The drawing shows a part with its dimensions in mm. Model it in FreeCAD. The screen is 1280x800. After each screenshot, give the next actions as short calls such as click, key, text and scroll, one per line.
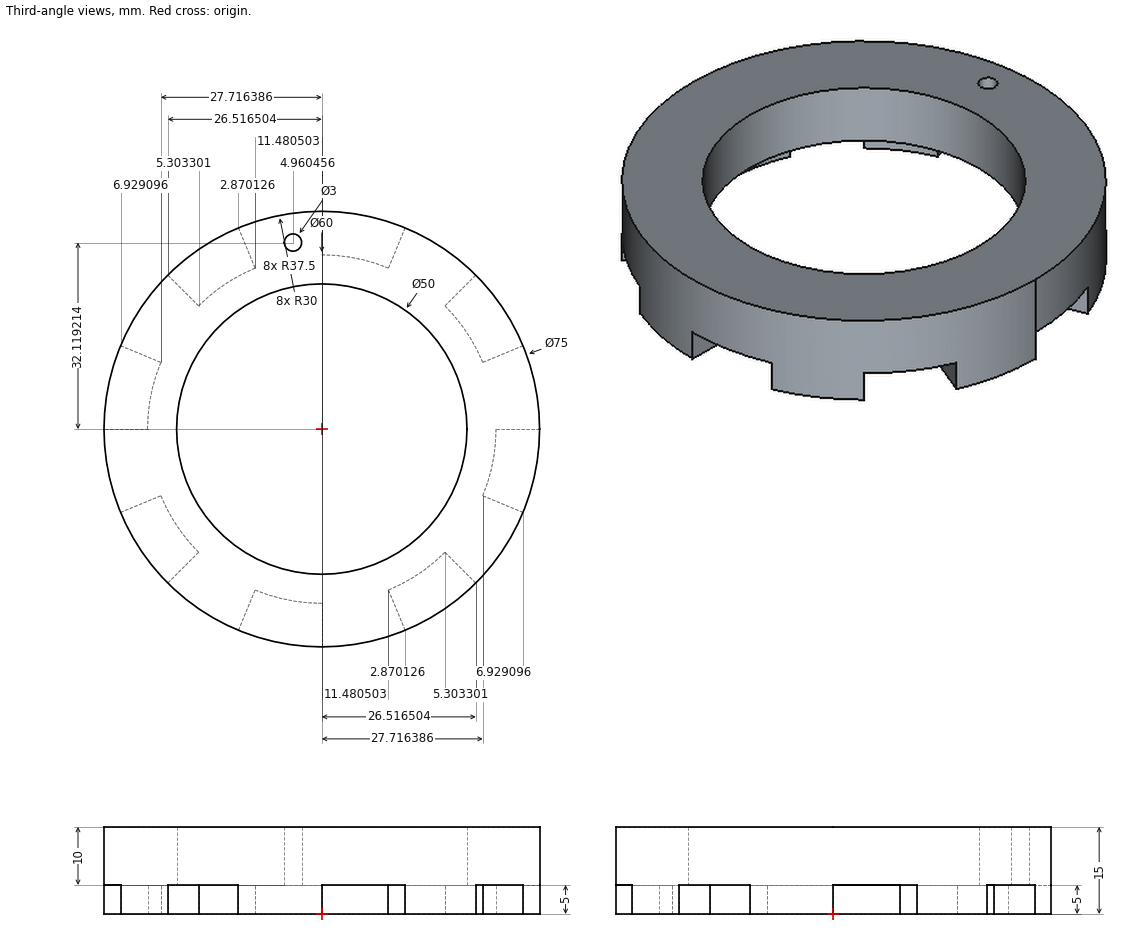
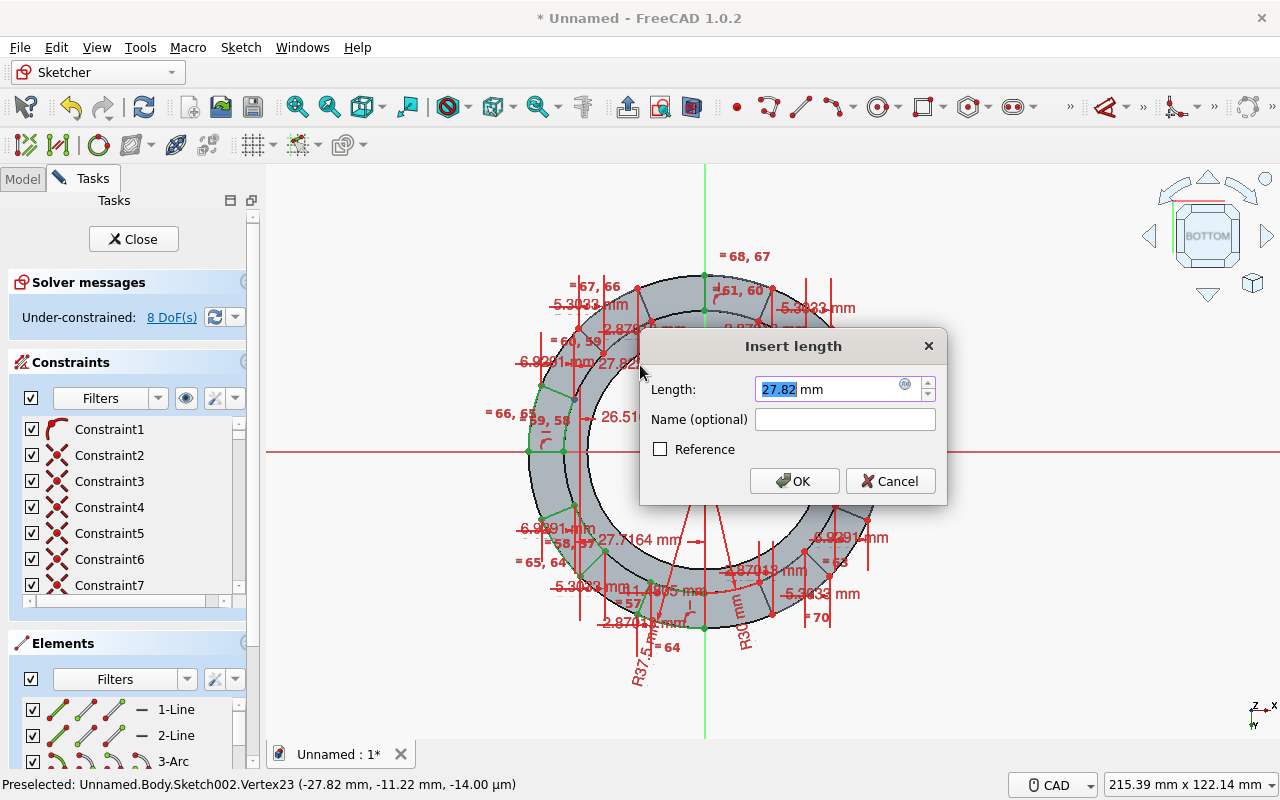
text(27.716386)
key(Return)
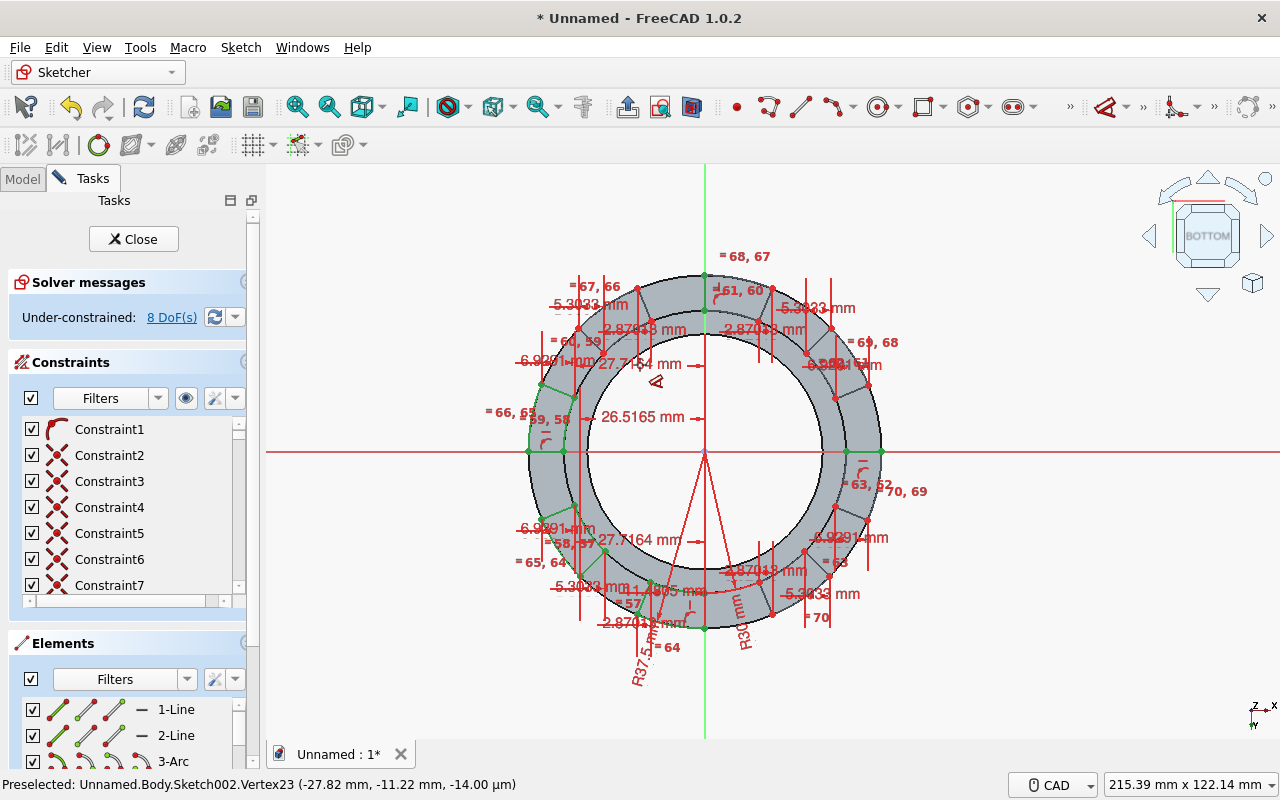
click(579, 329)
click(671, 295)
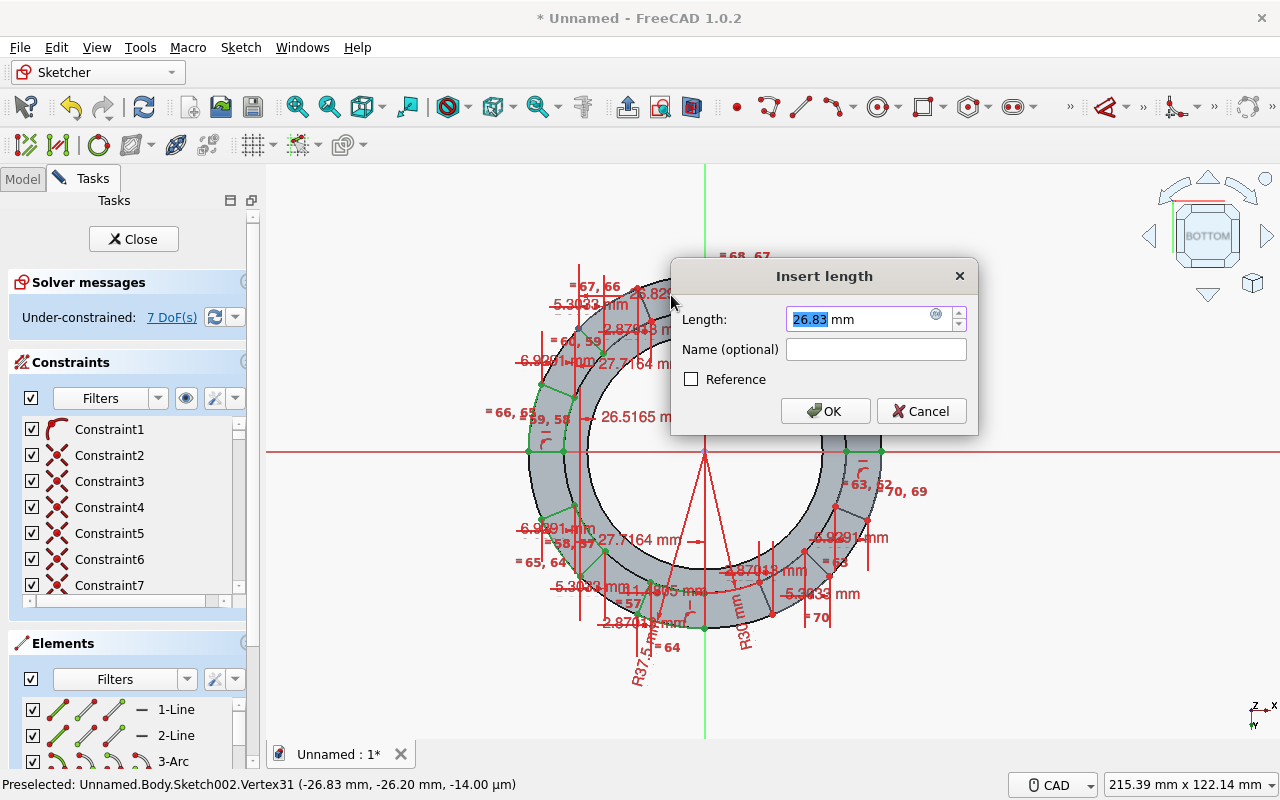
text(26.516504)
key(Return)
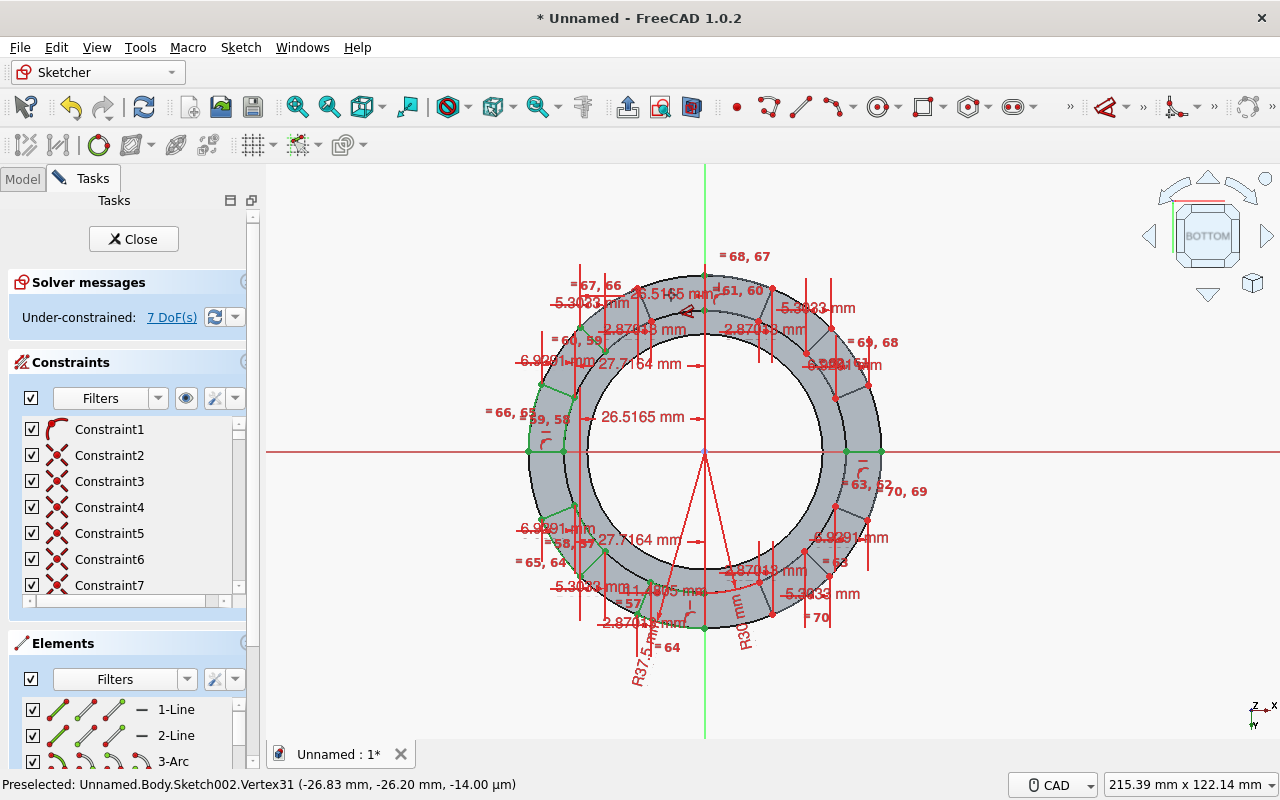
click(651, 321)
click(678, 486)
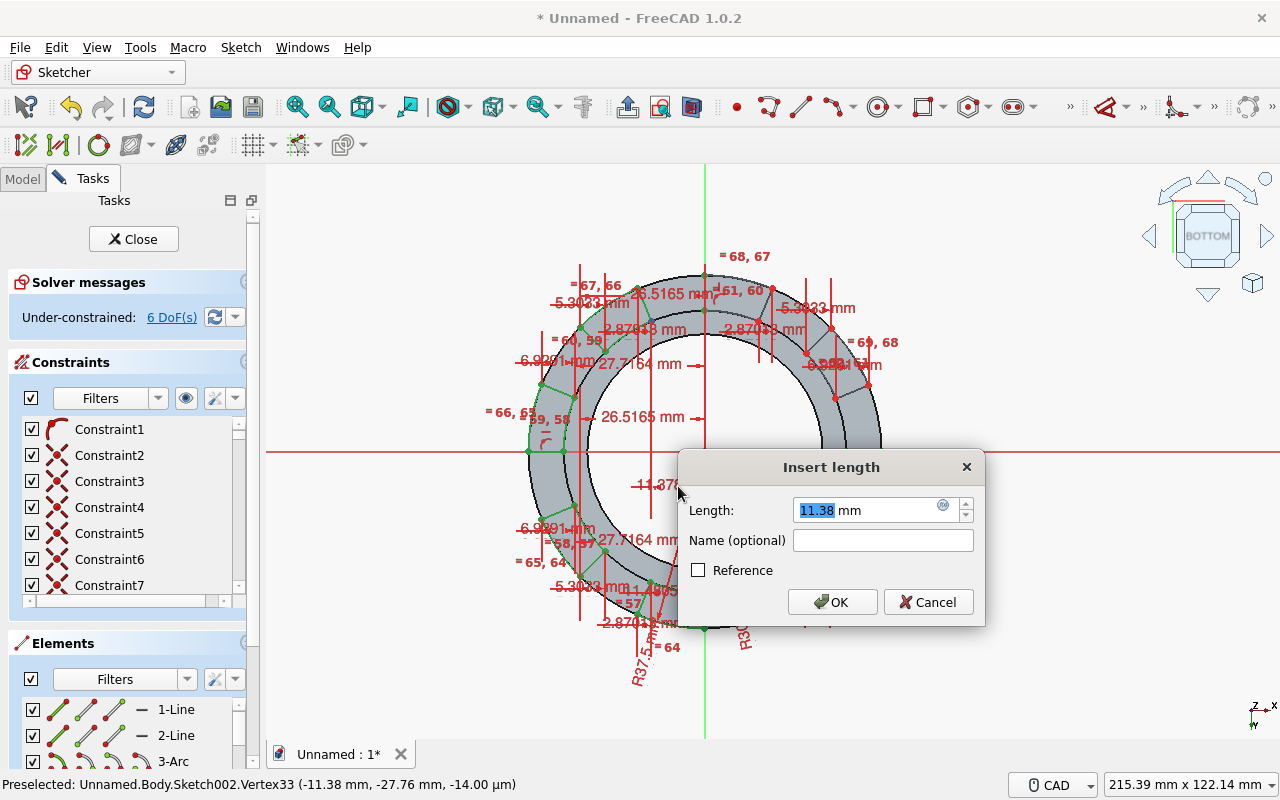
text(11.480503)
key(Return)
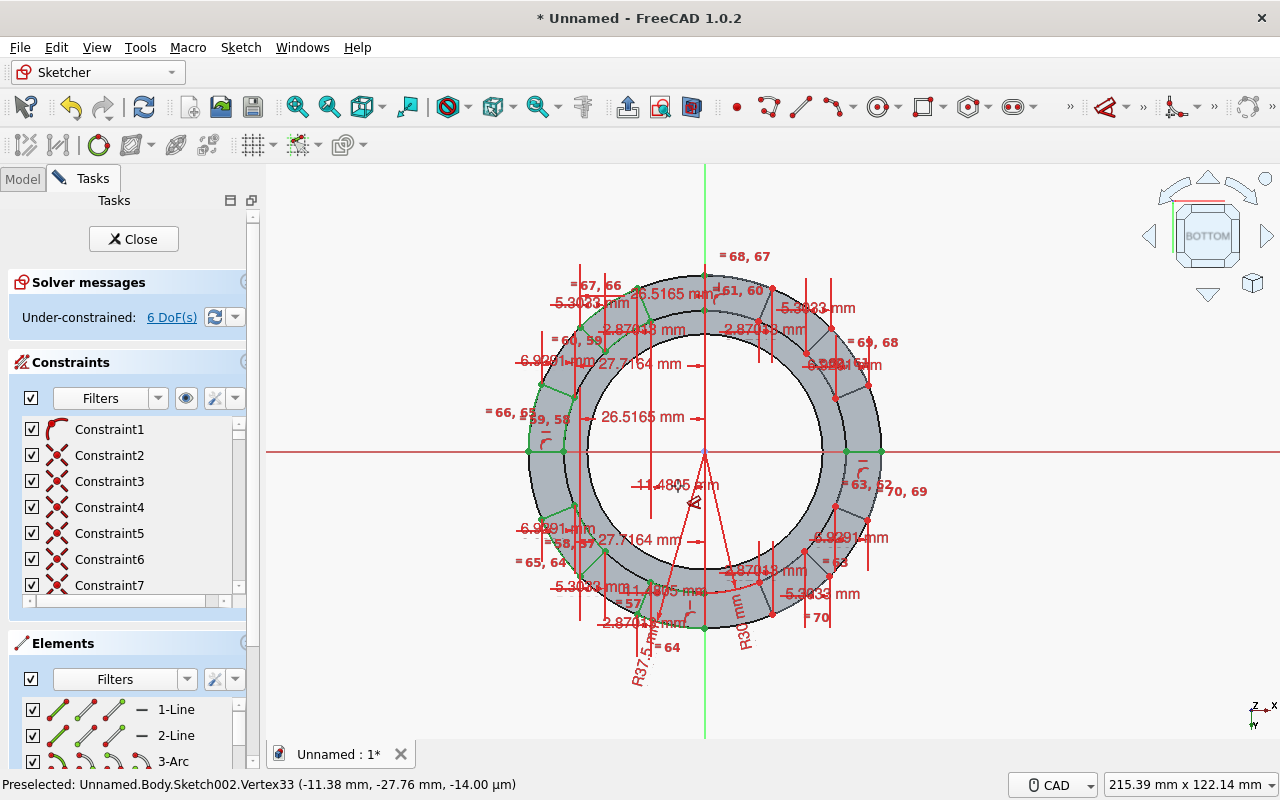
click(759, 321)
click(751, 486)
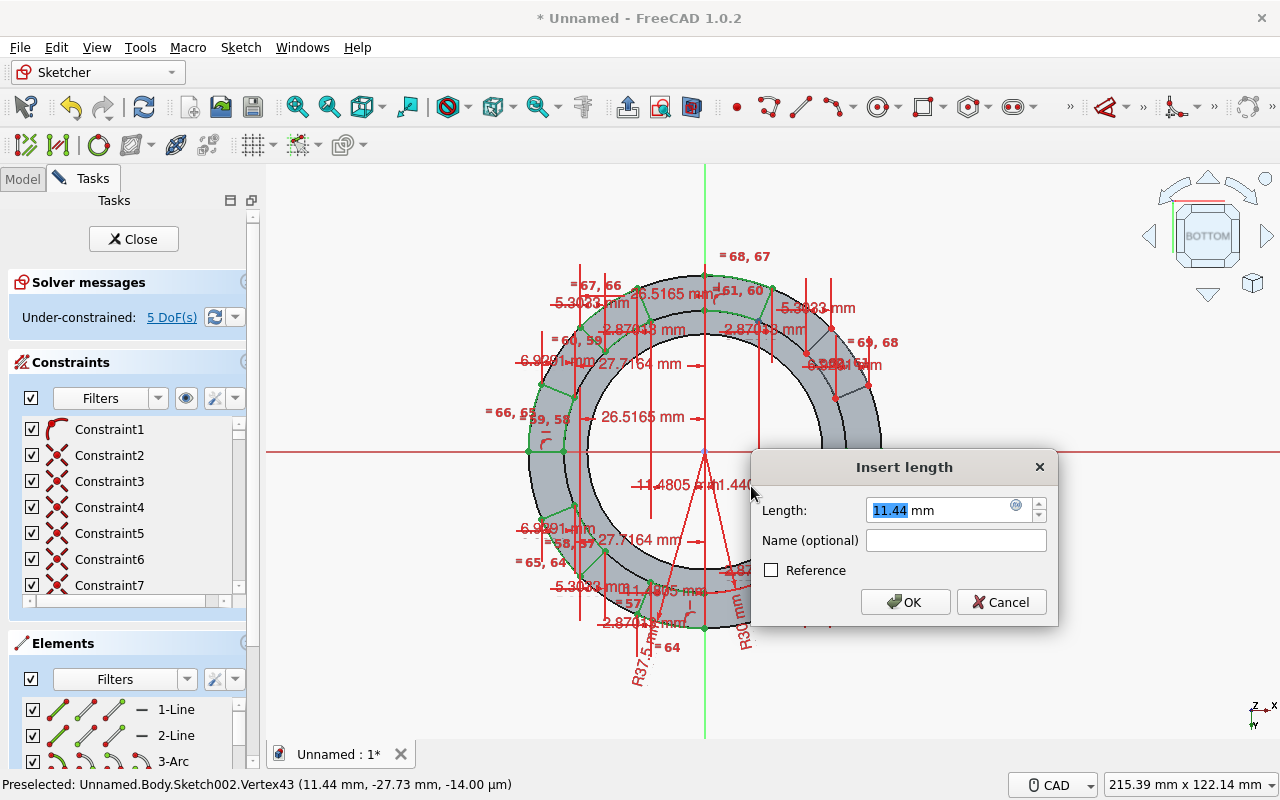
text(11.480503)
key(Return)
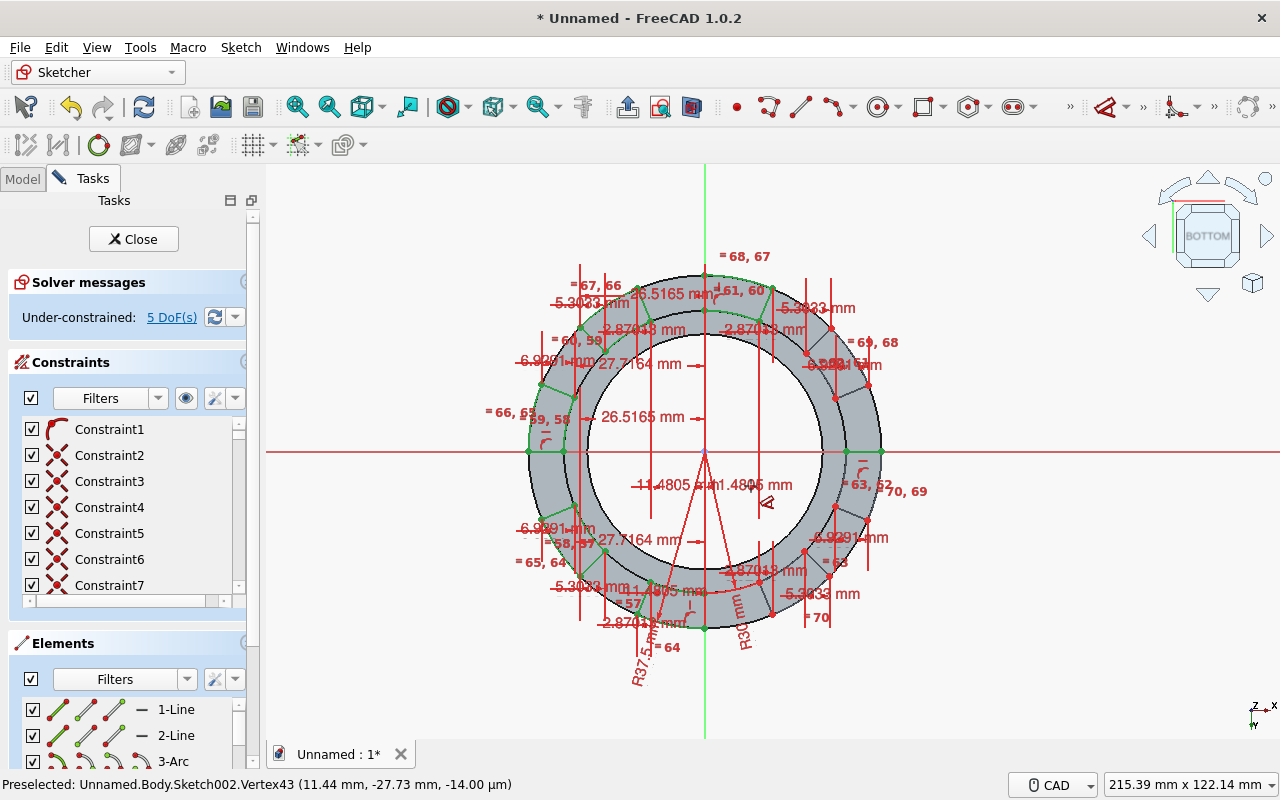
click(831, 328)
click(768, 270)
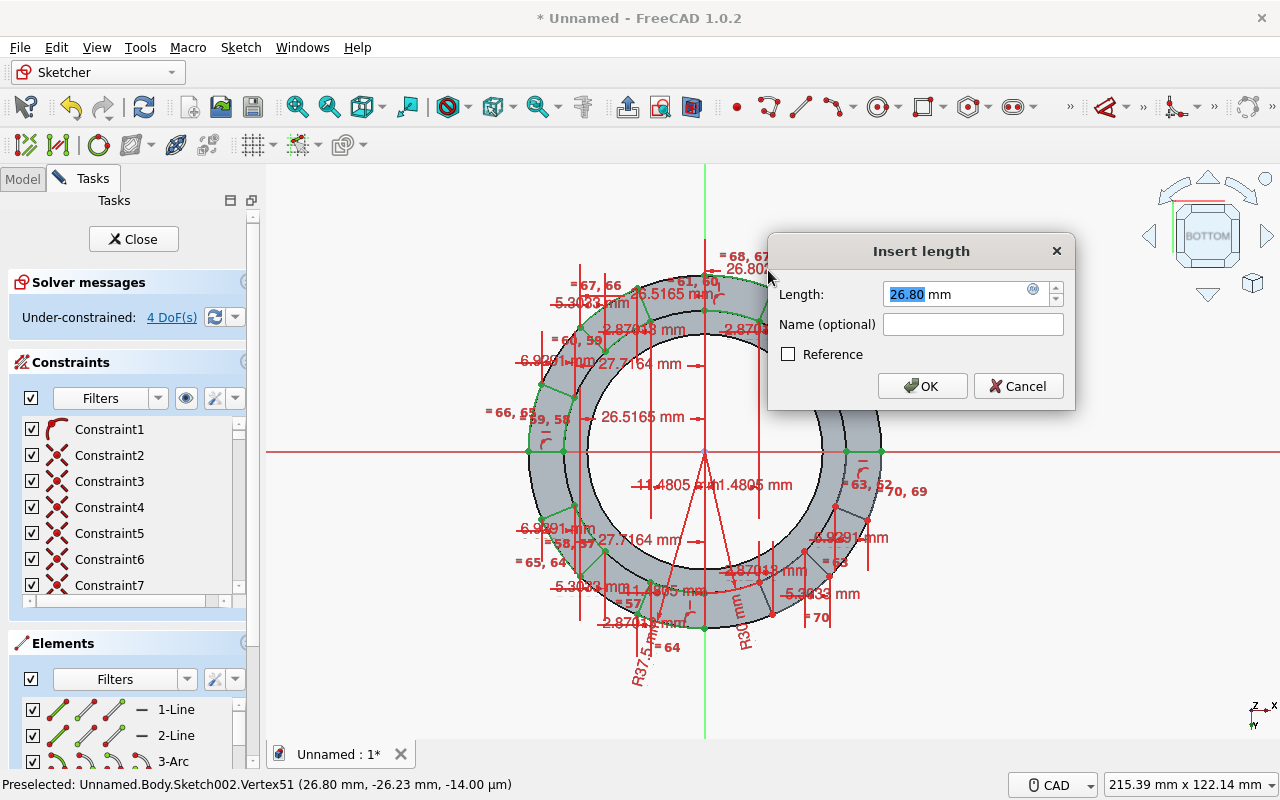
text(26.516504)
key(Return)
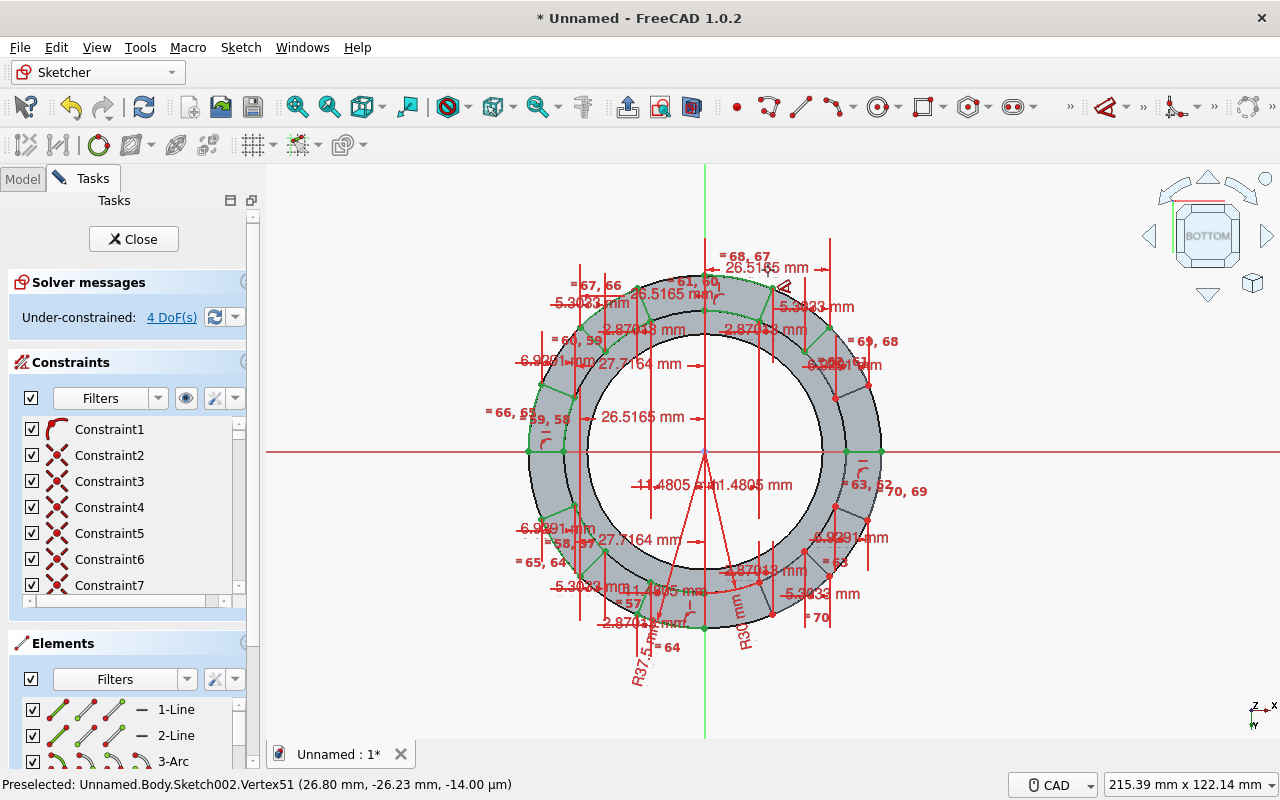
click(836, 399)
click(770, 365)